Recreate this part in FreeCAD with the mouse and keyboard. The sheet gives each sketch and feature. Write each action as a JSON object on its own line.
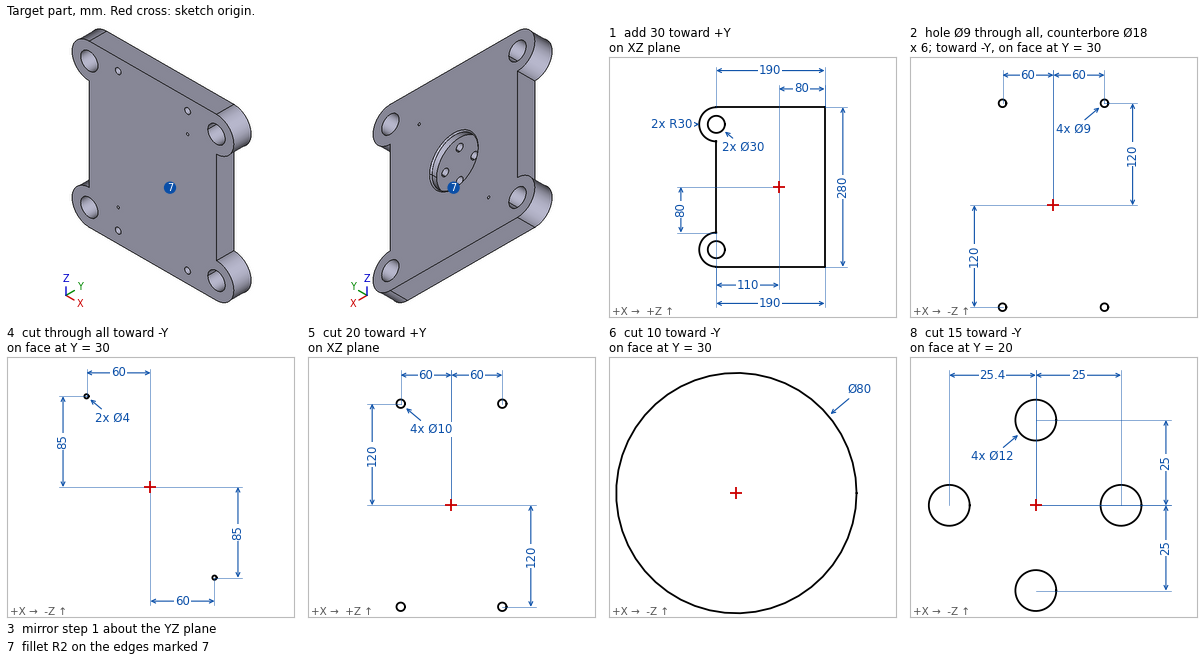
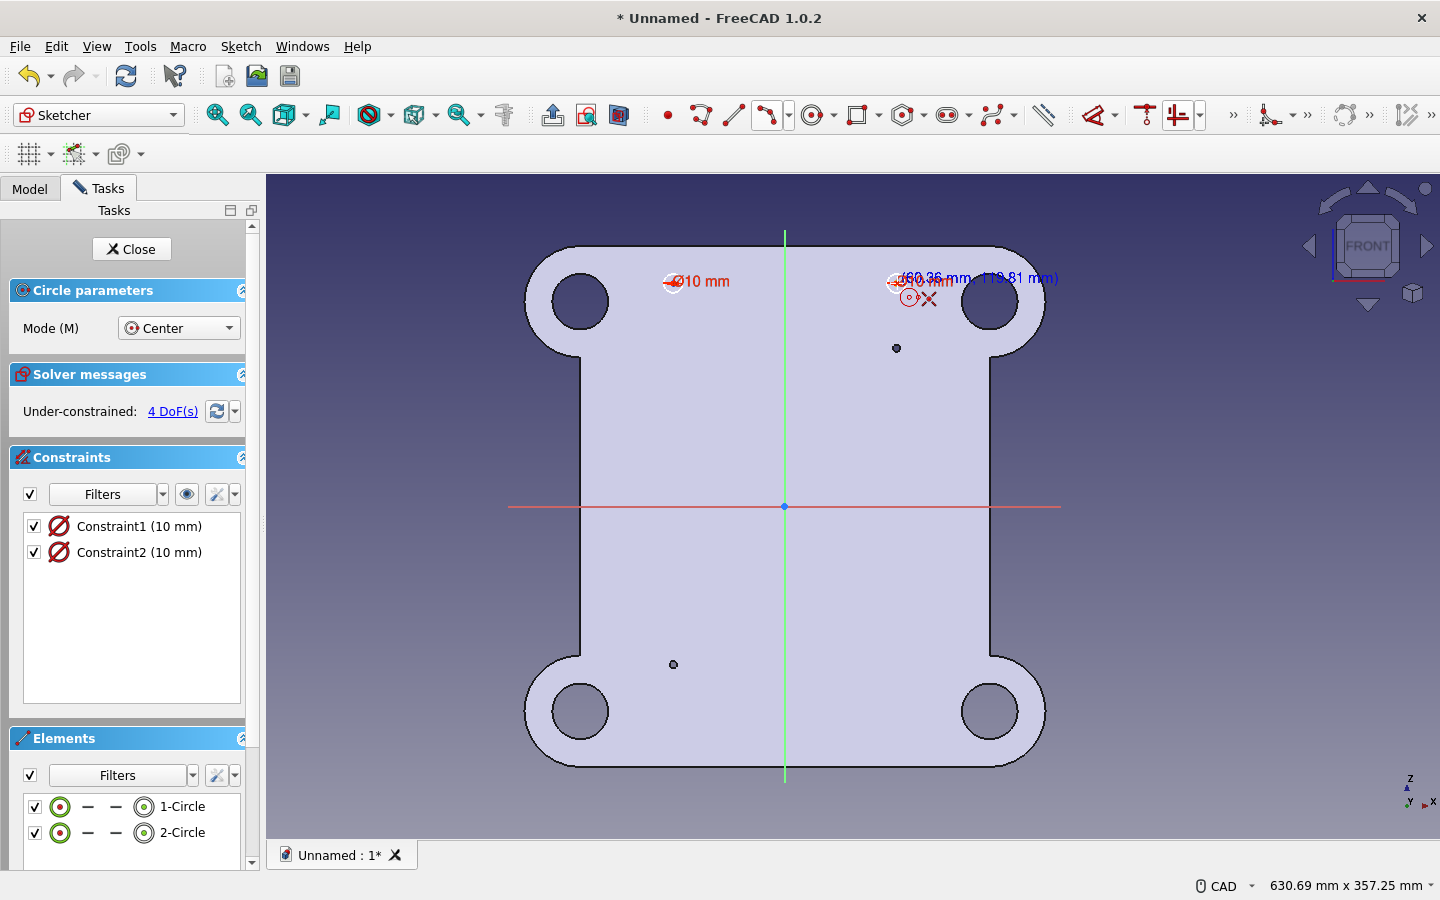
{"action": "scroll", "coordinate": [897, 730], "scroll_direction": "up", "scroll_amount": 5}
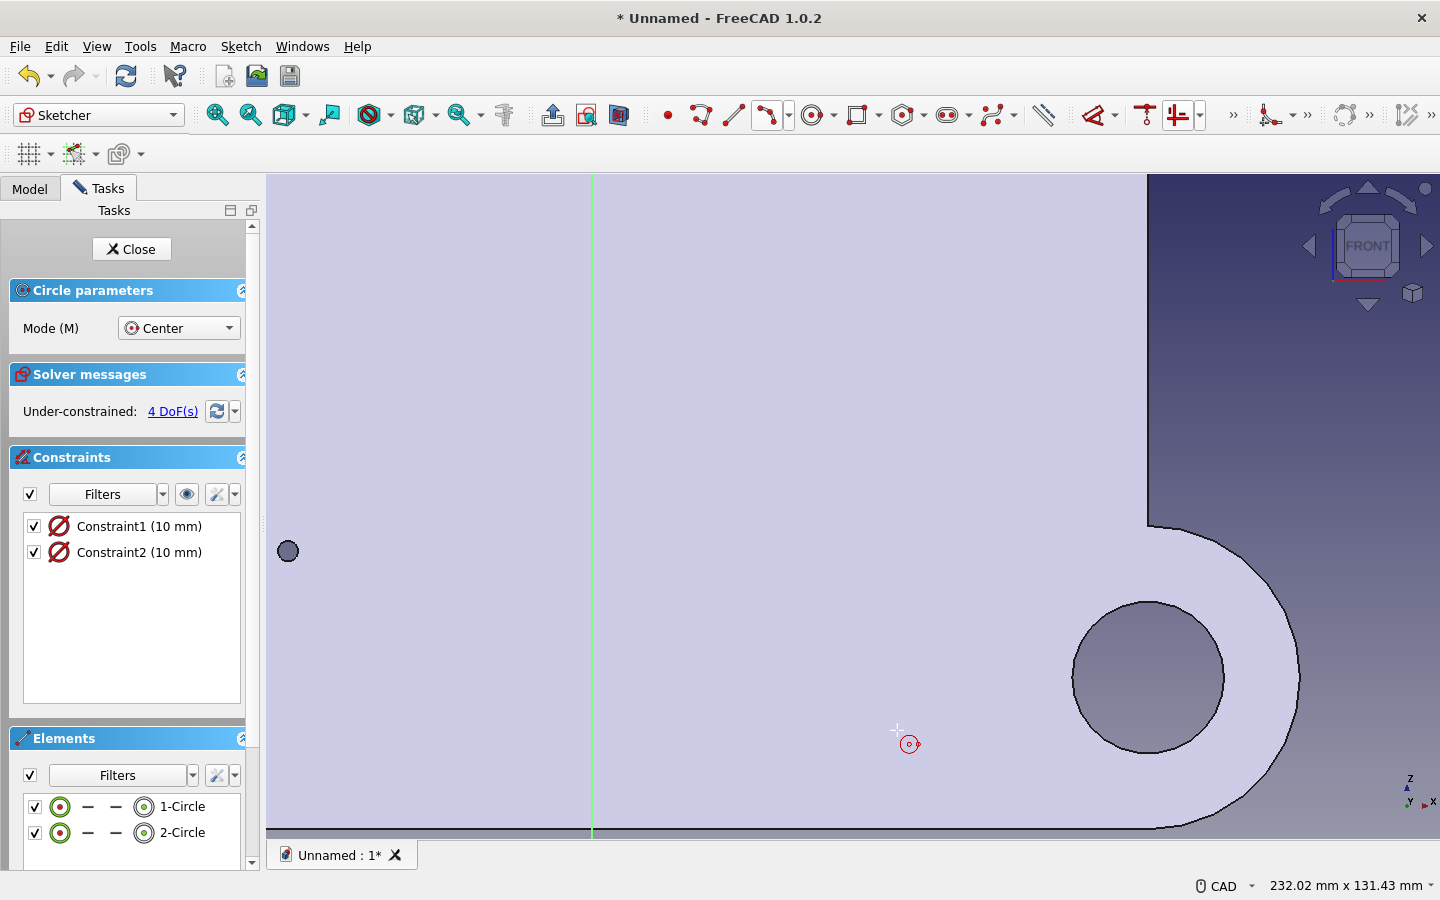
{"action": "left_click", "coordinate": [895, 728]}
{"action": "mouse_move", "coordinate": [913, 710]}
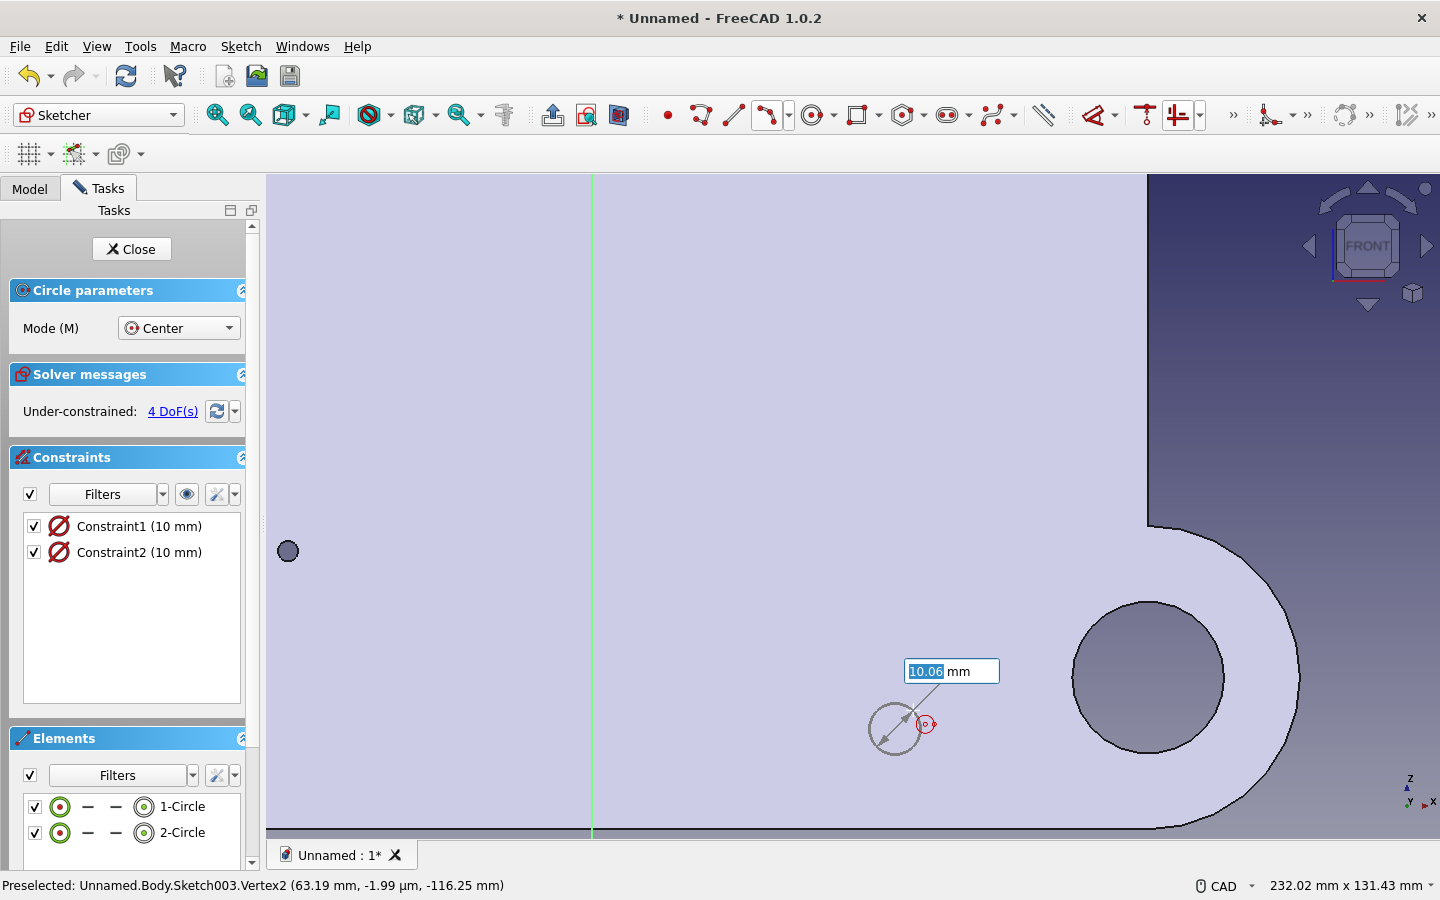
{"action": "type", "text": "10"}
{"action": "key", "text": "Return"}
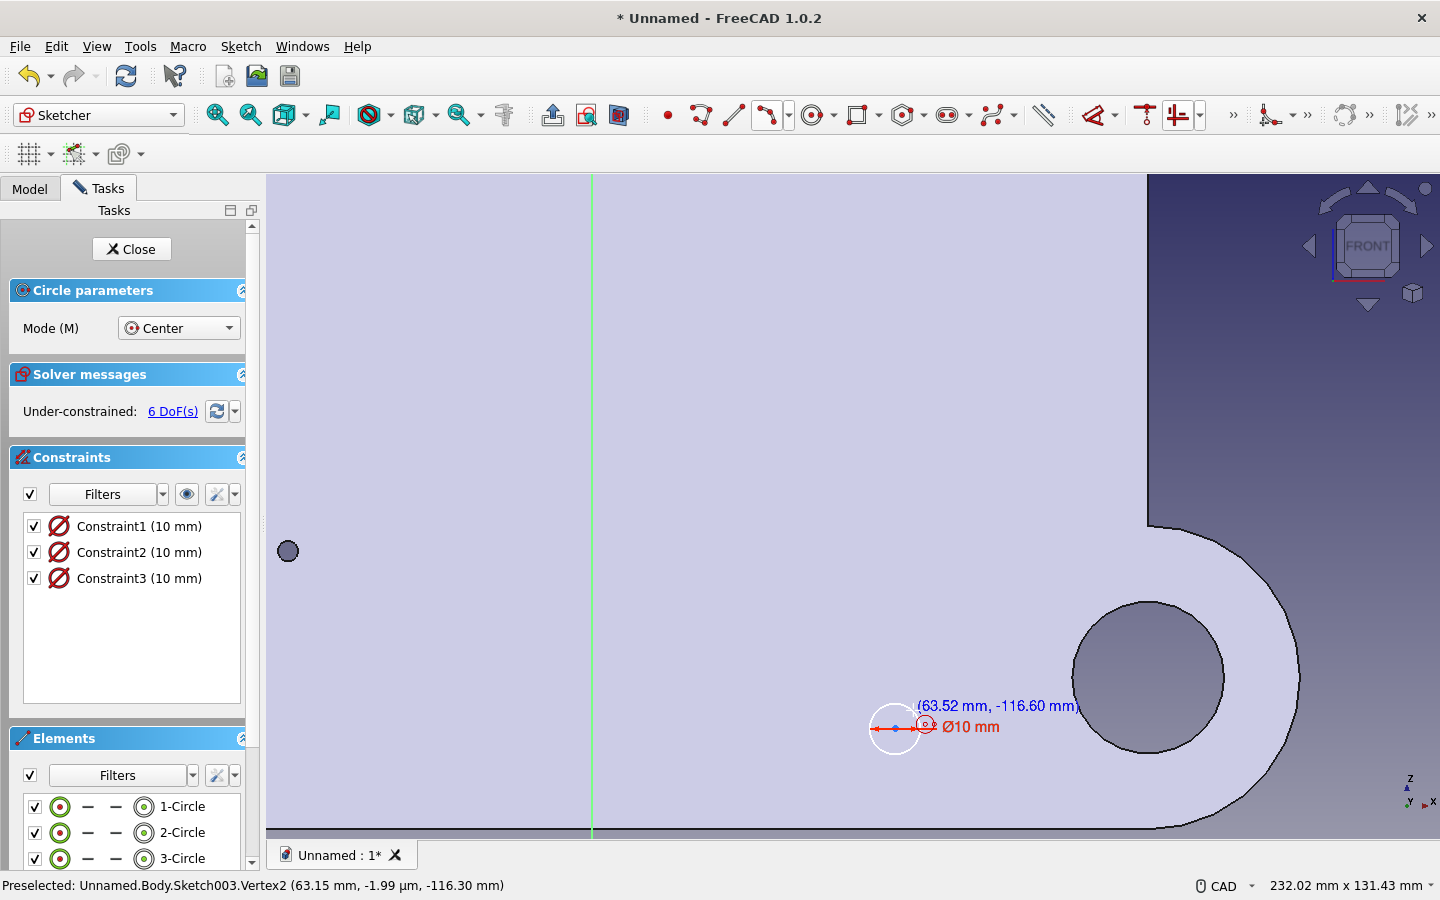
{"action": "scroll", "coordinate": [897, 731], "scroll_direction": "down", "scroll_amount": 5}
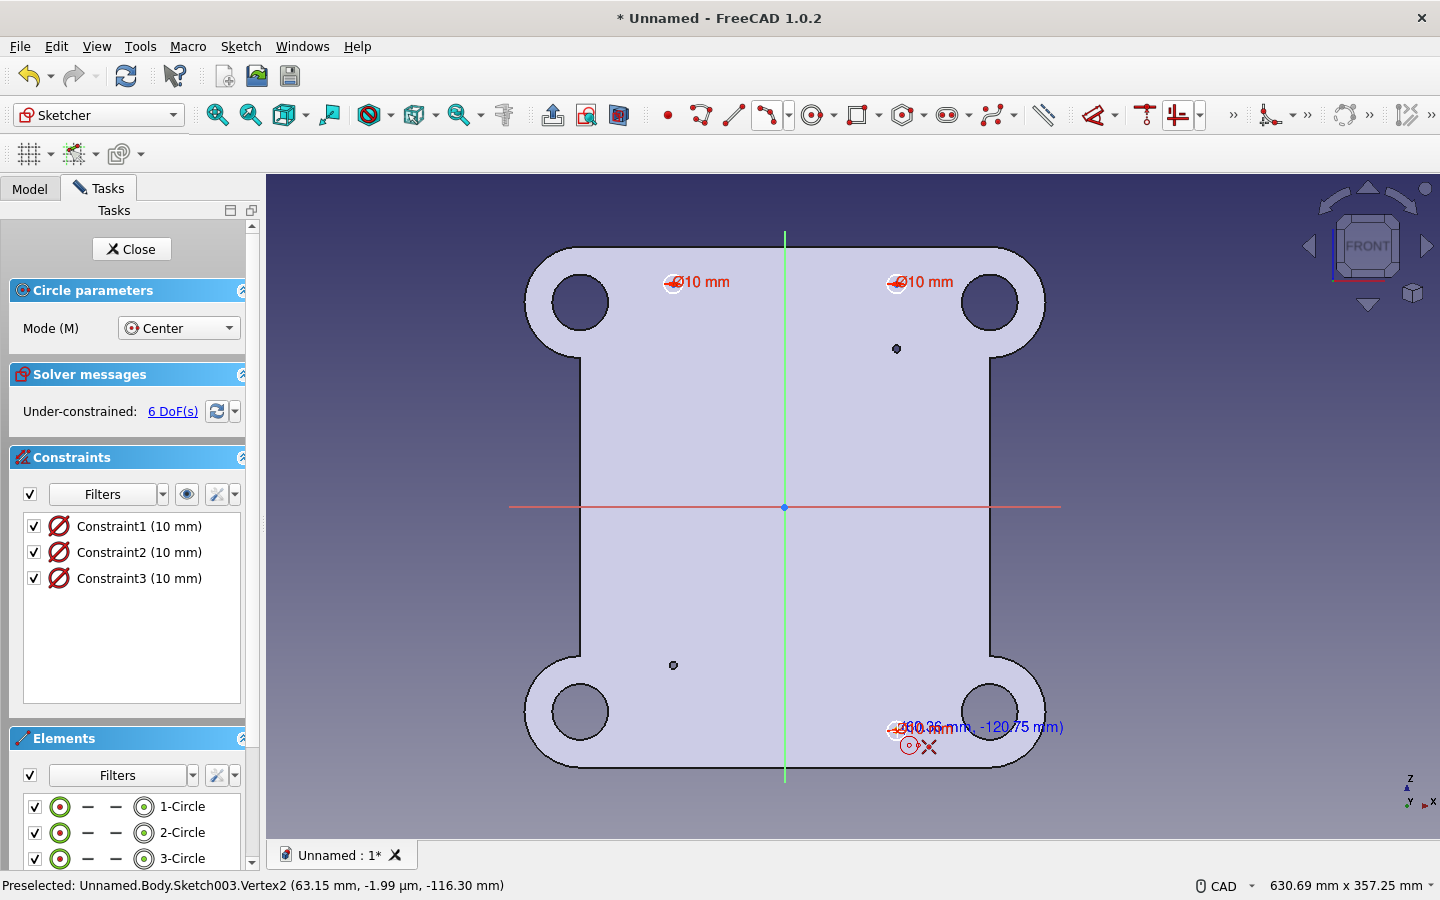
{"action": "scroll", "coordinate": [673, 731], "scroll_direction": "up", "scroll_amount": 5}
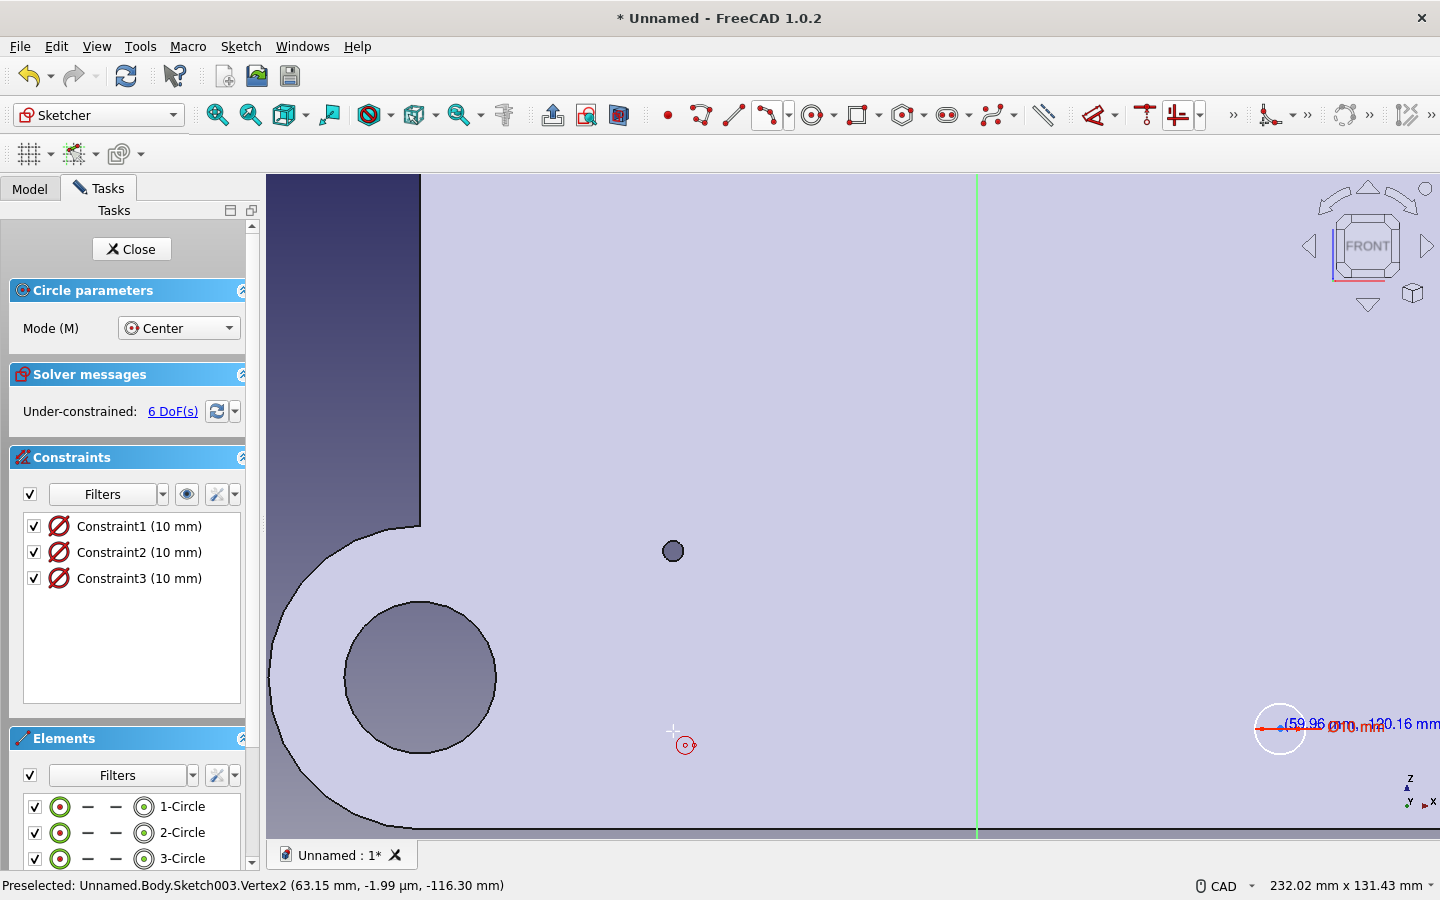
{"action": "left_click", "coordinate": [673, 728]}
{"action": "mouse_move", "coordinate": [691, 710]}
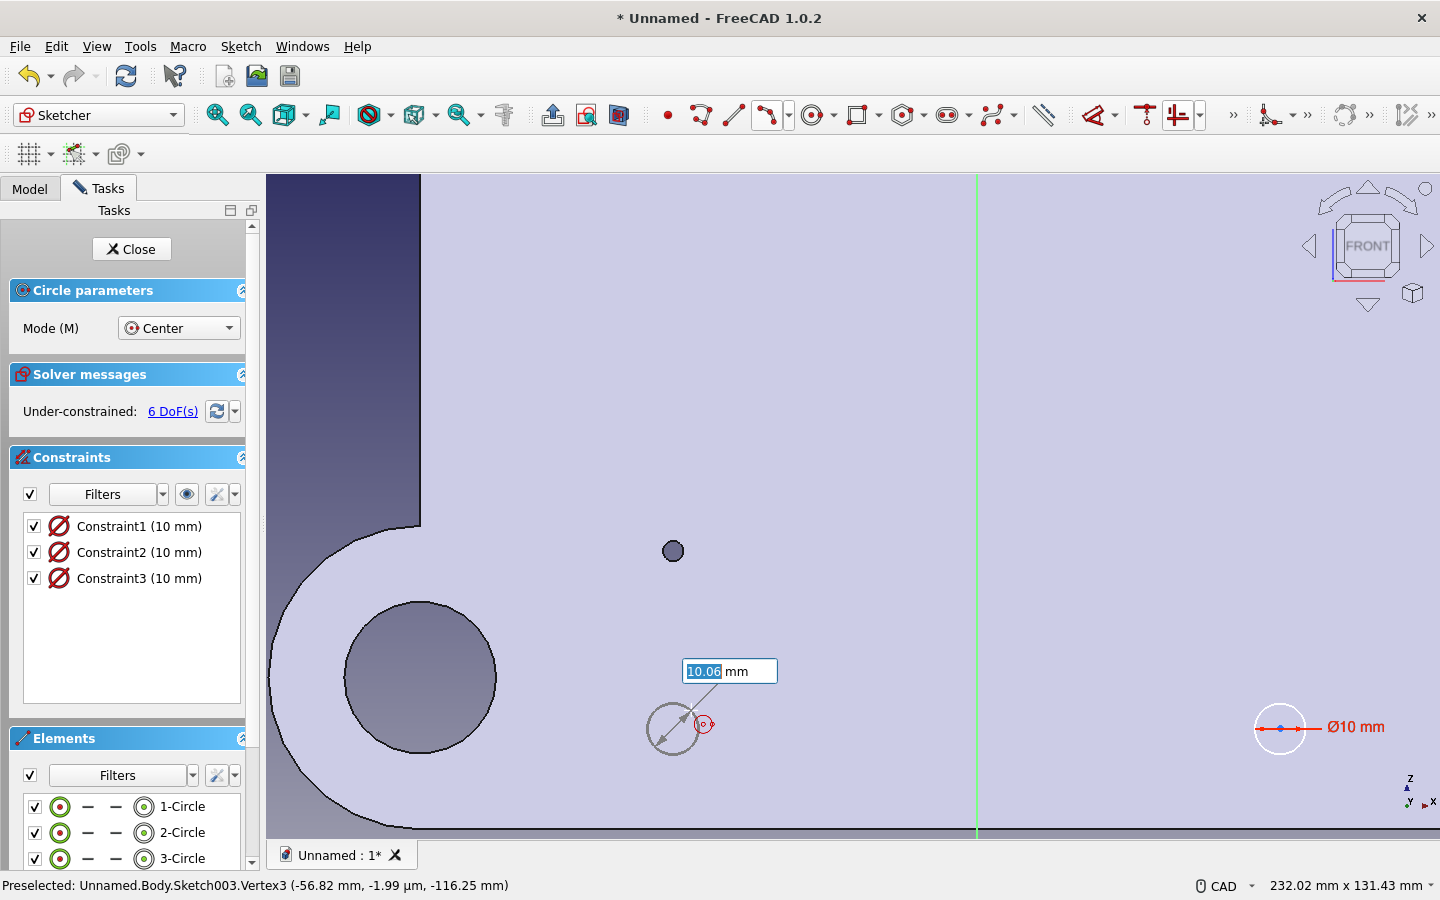
{"action": "type", "text": "10"}
{"action": "key", "text": "Return"}
{"action": "key", "text": "Escape"}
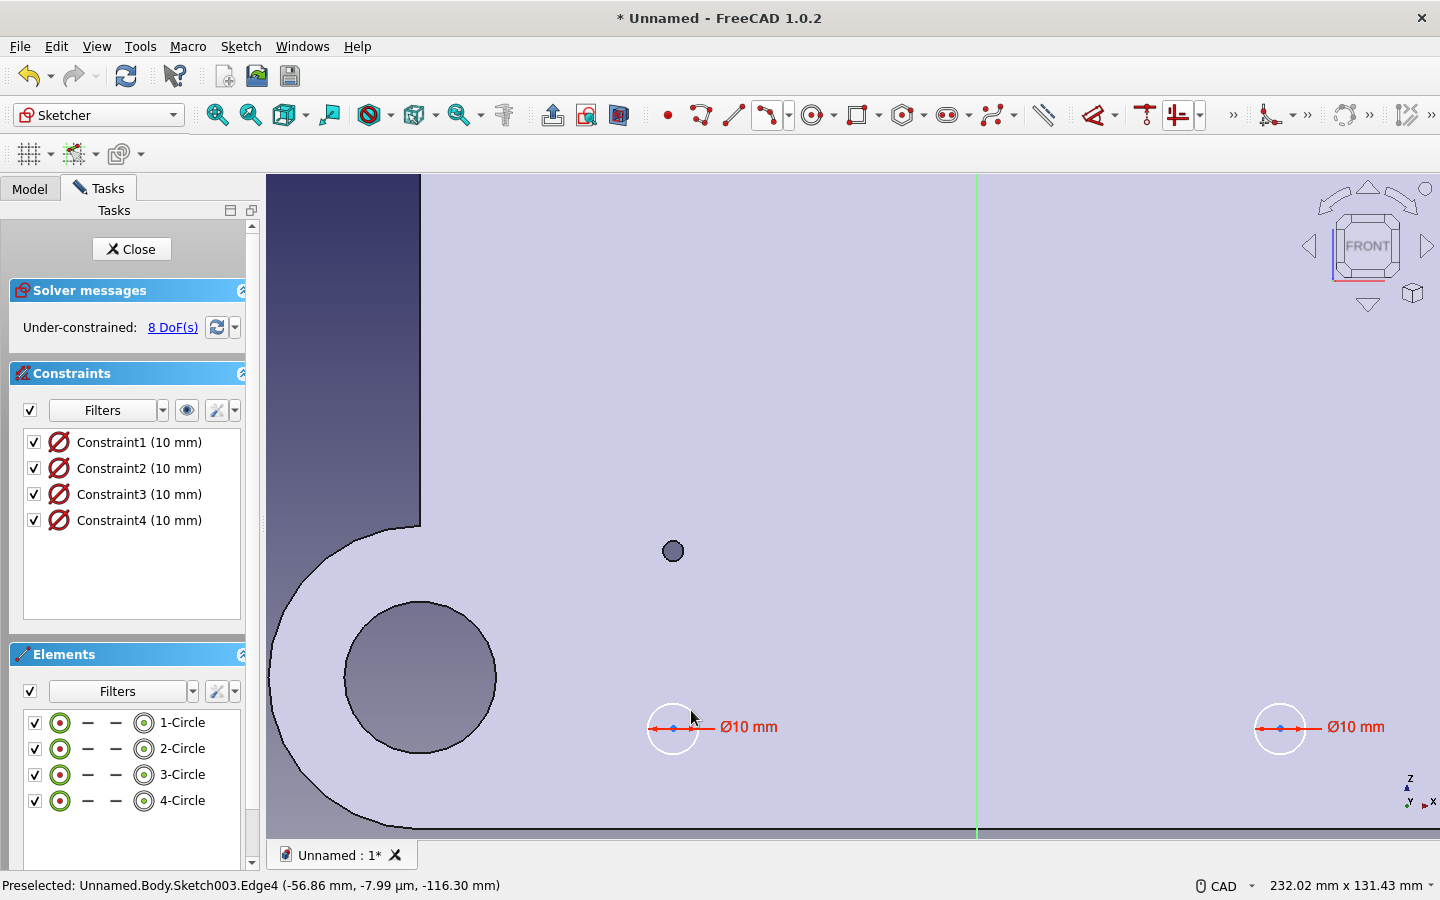
{"action": "scroll", "coordinate": [673, 731], "scroll_direction": "down", "scroll_amount": 5}